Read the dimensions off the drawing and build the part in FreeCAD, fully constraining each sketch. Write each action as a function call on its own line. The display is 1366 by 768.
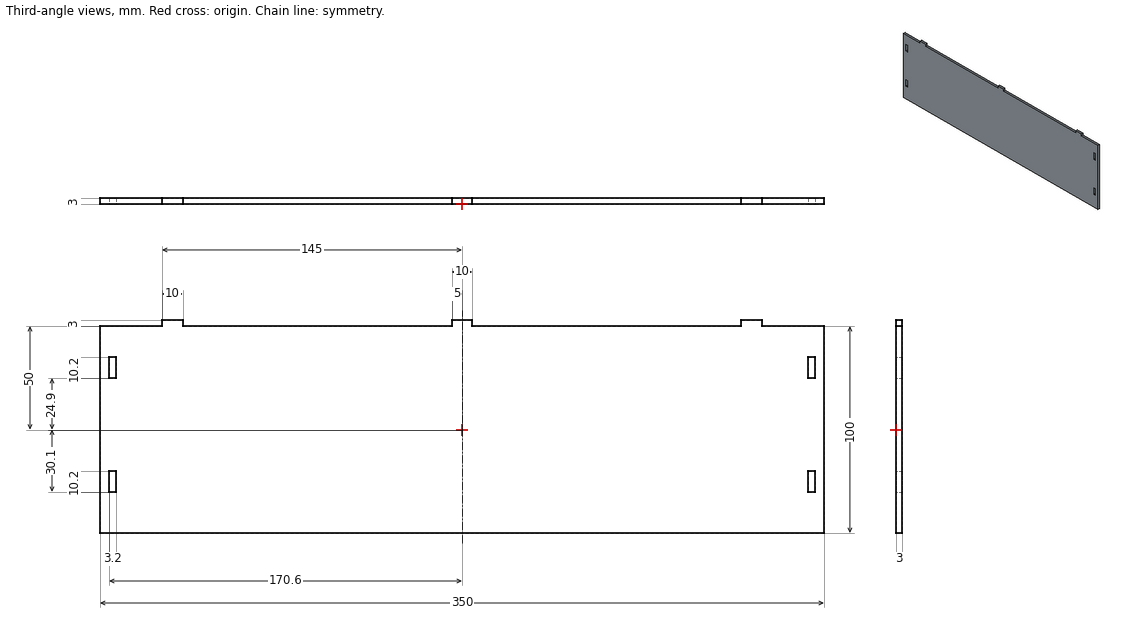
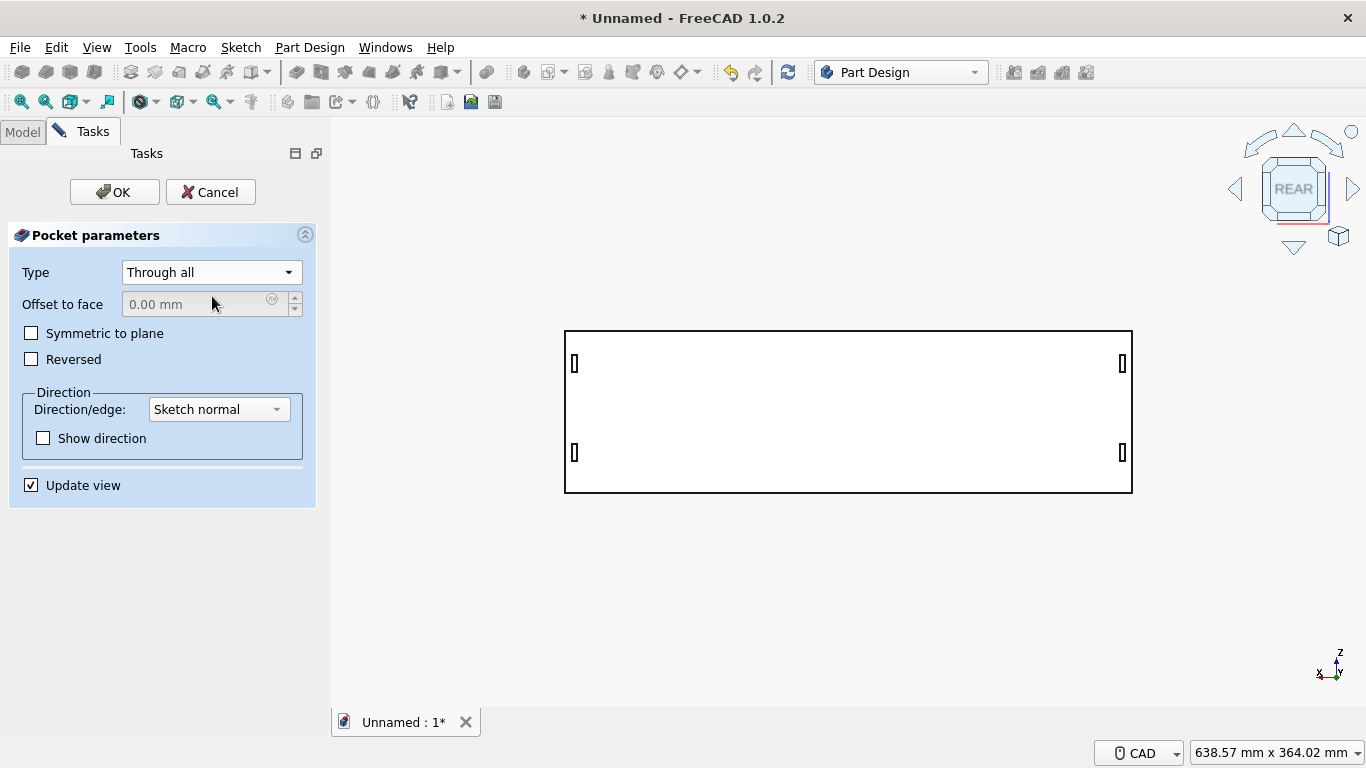
click(115, 192)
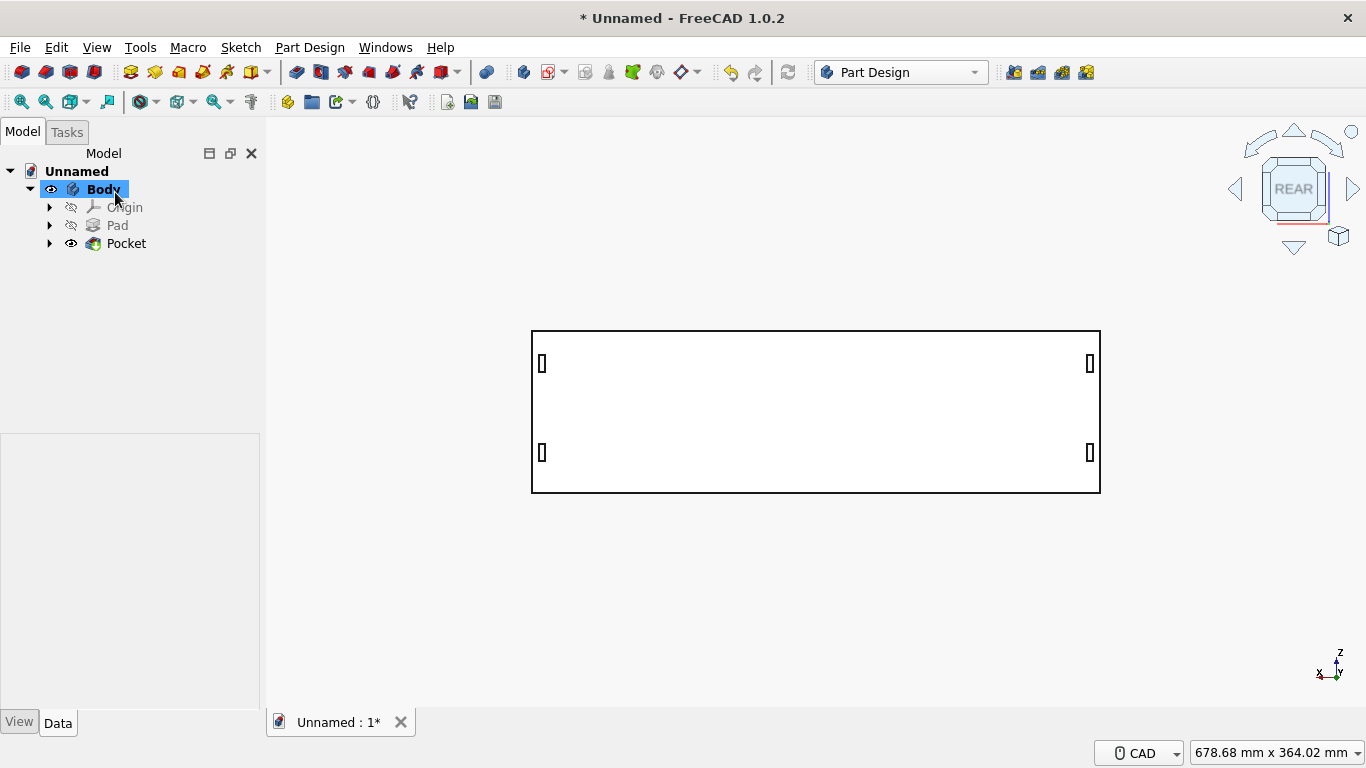
click(654, 411)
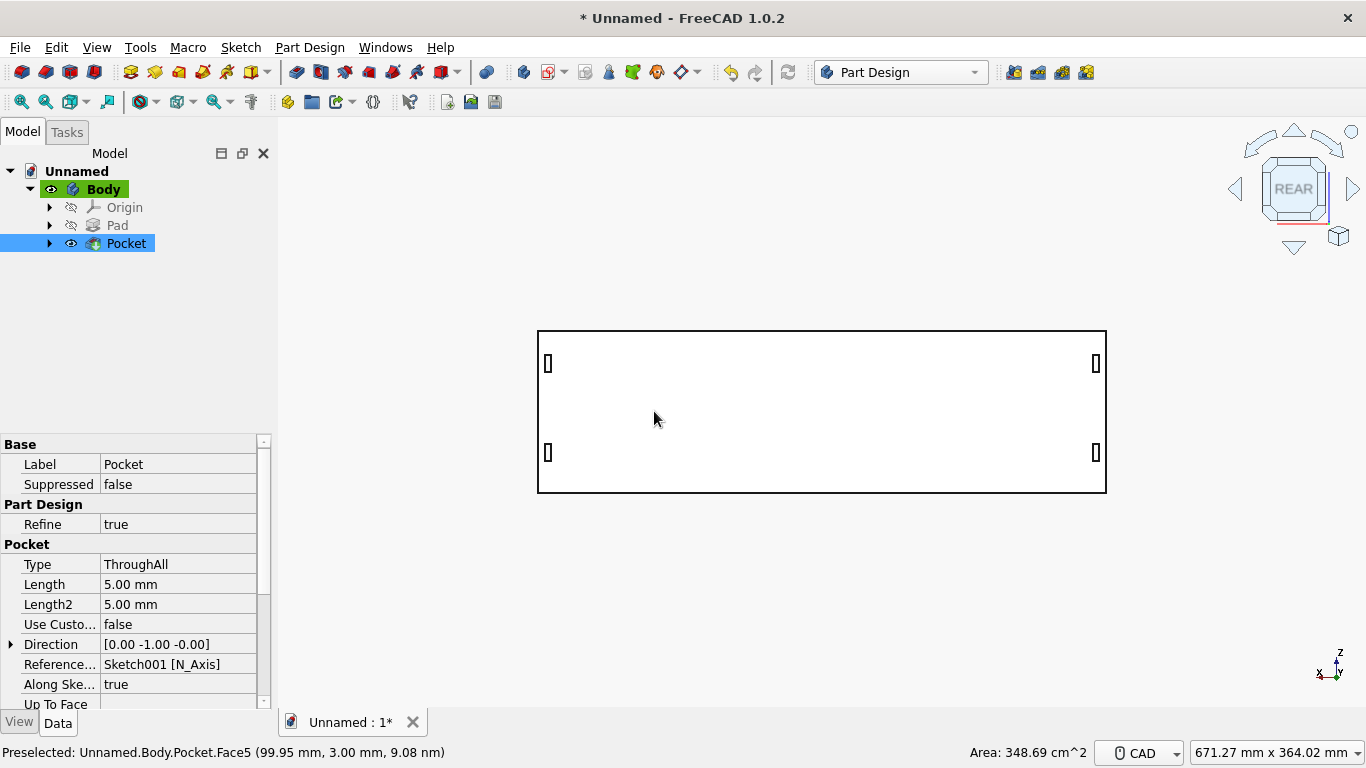
click(548, 72)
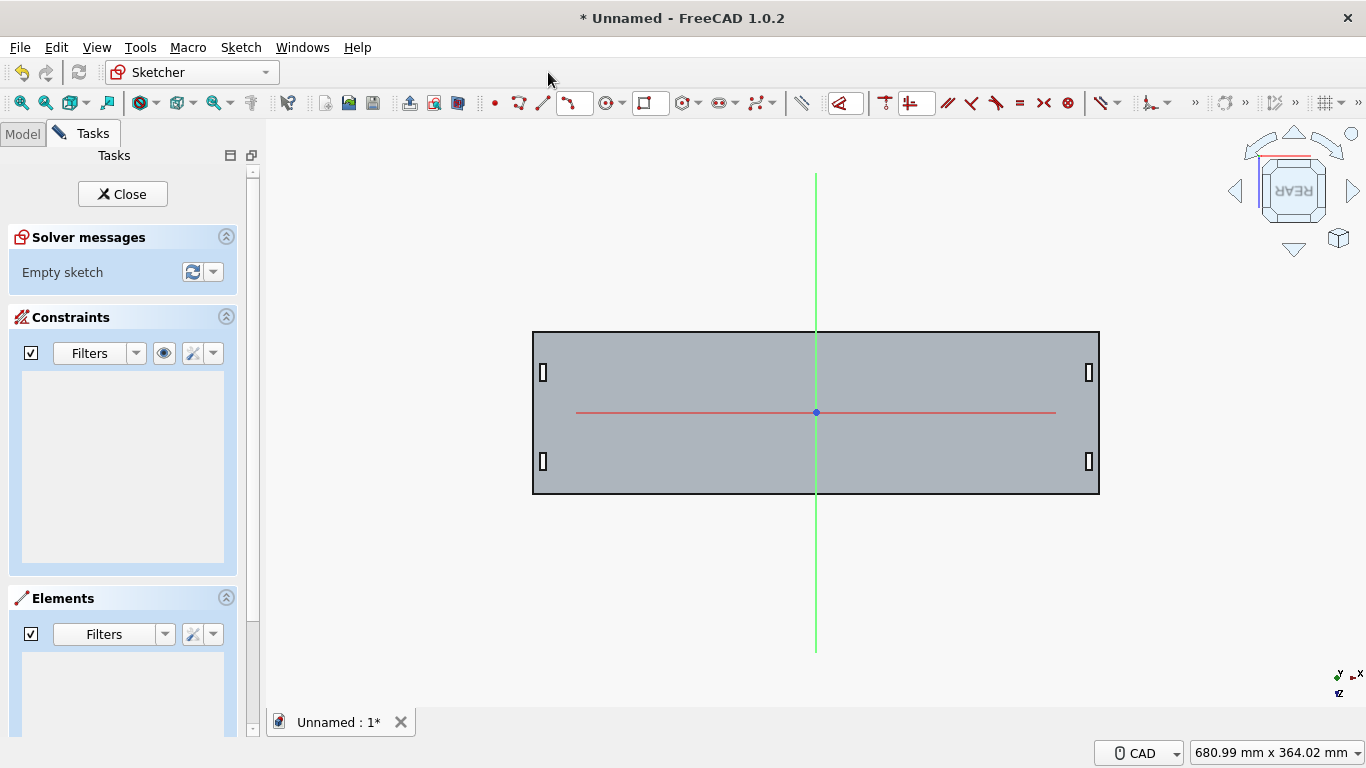
scroll(955, 543, up, 2)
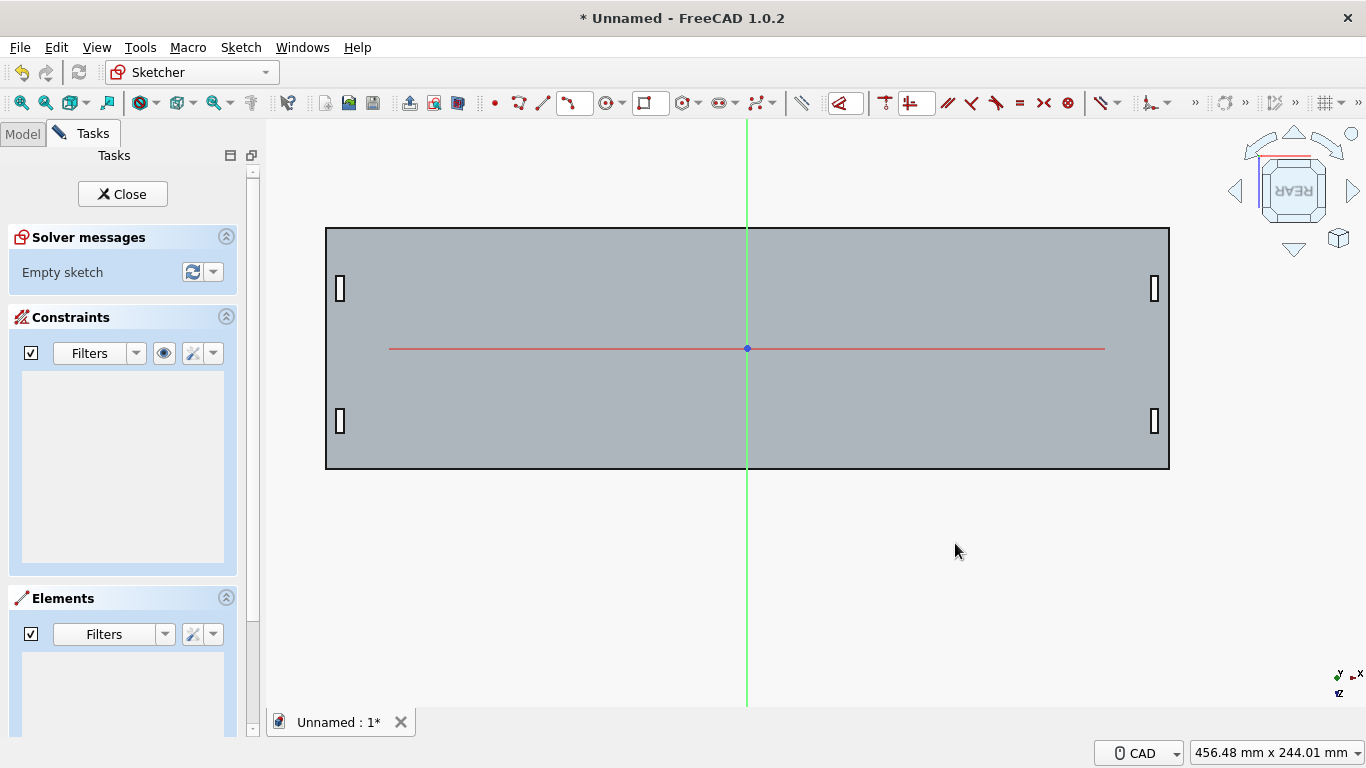
key(g)
key(r)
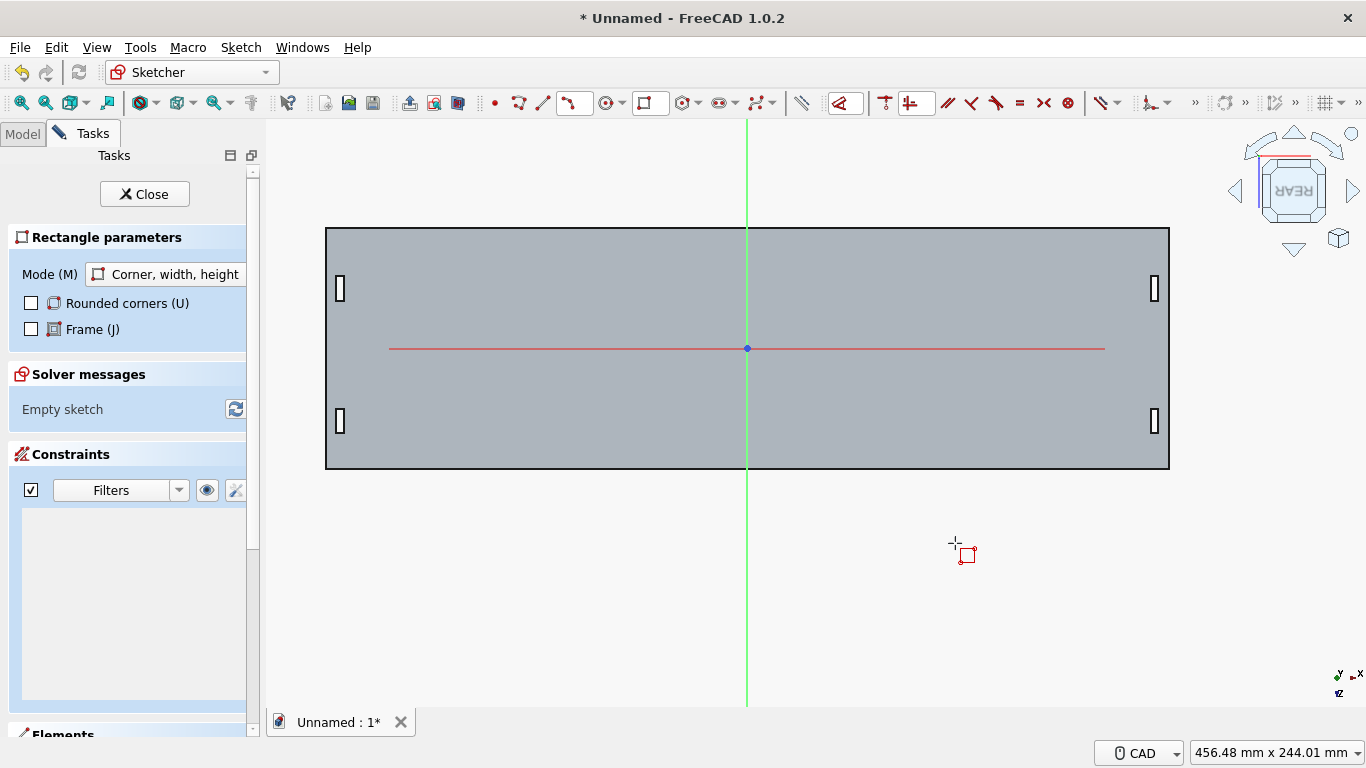
scroll(398, 469, up, 4)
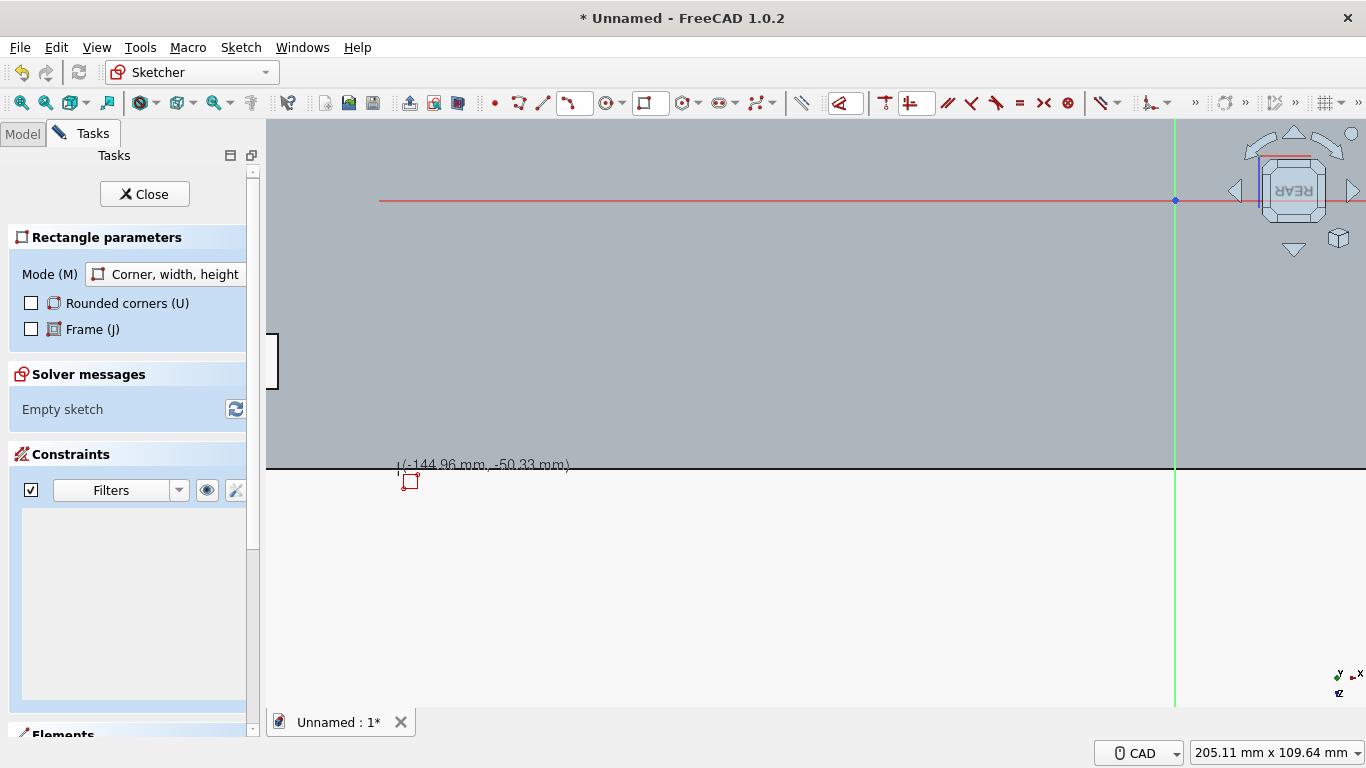
click(398, 469)
click(451, 485)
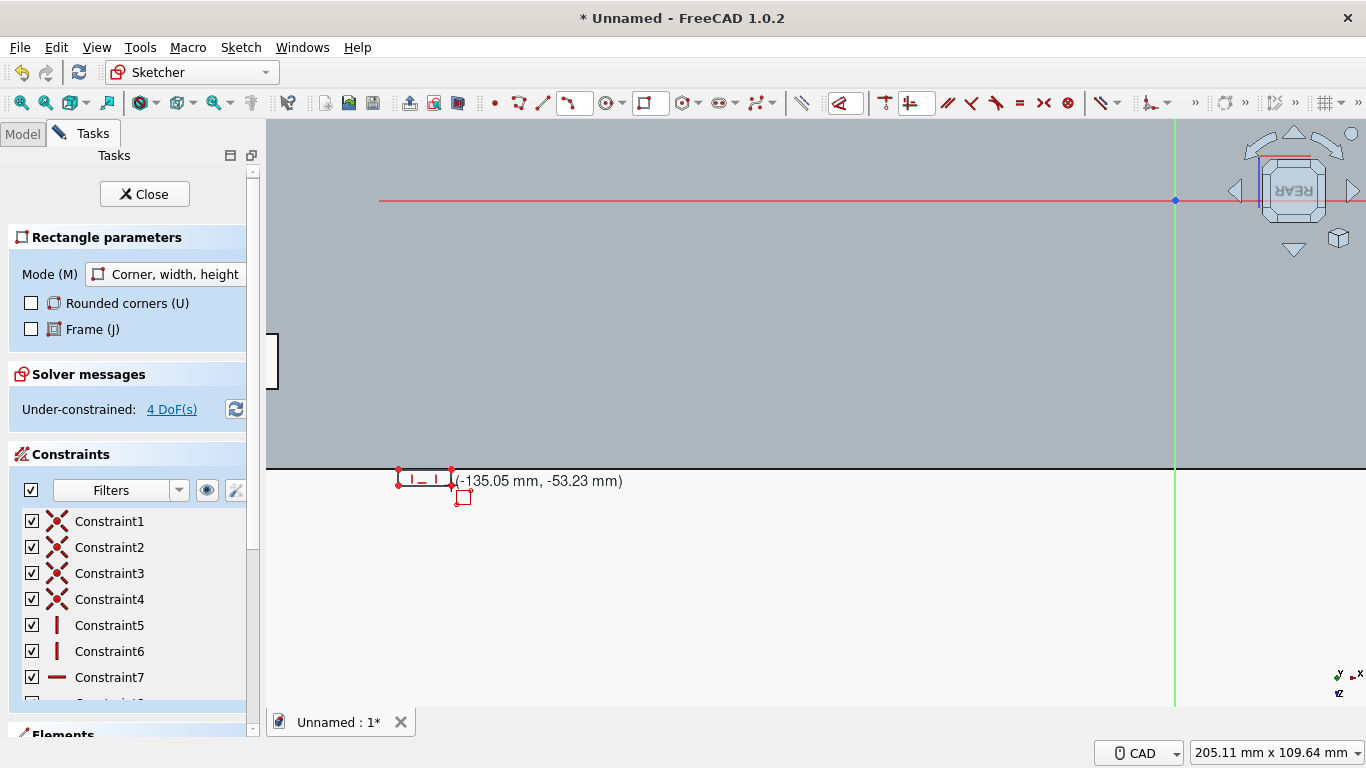
click(1148, 469)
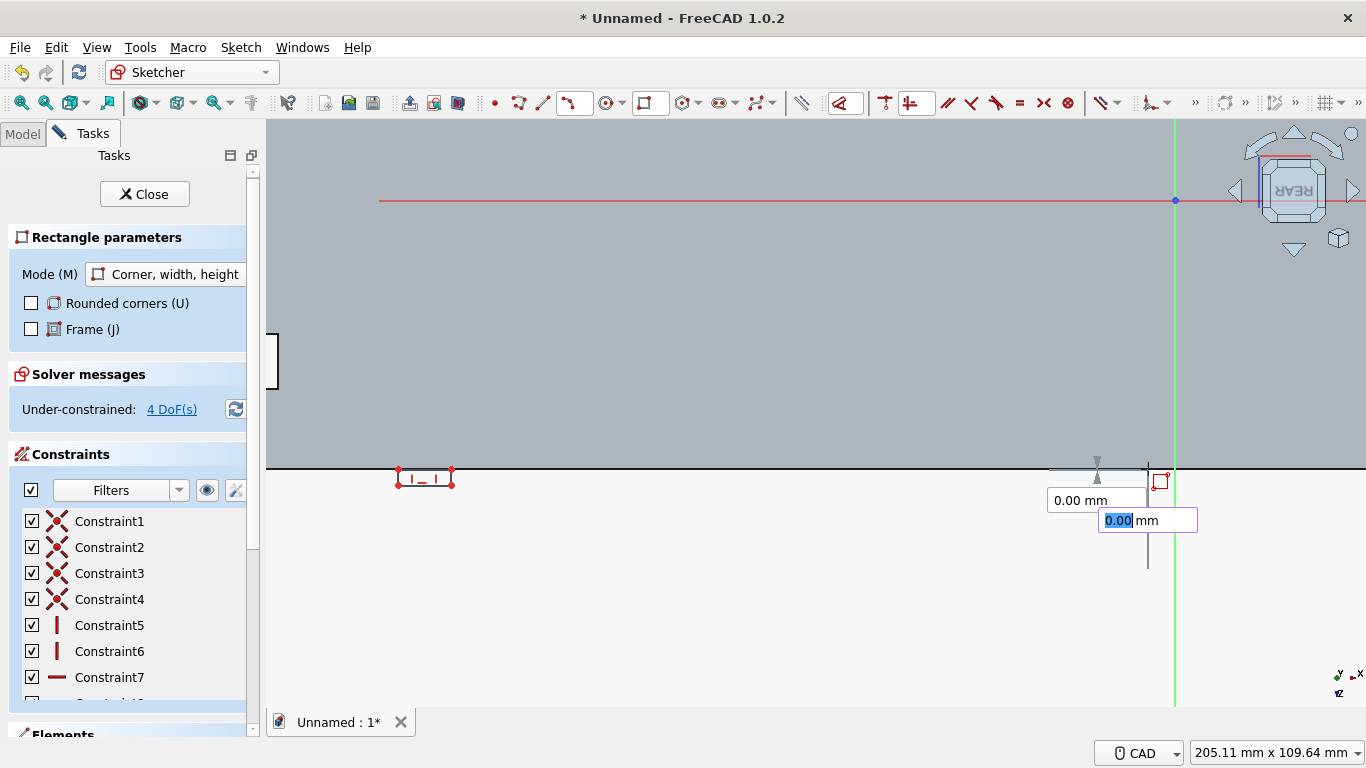
scroll(398, 470, down, 4)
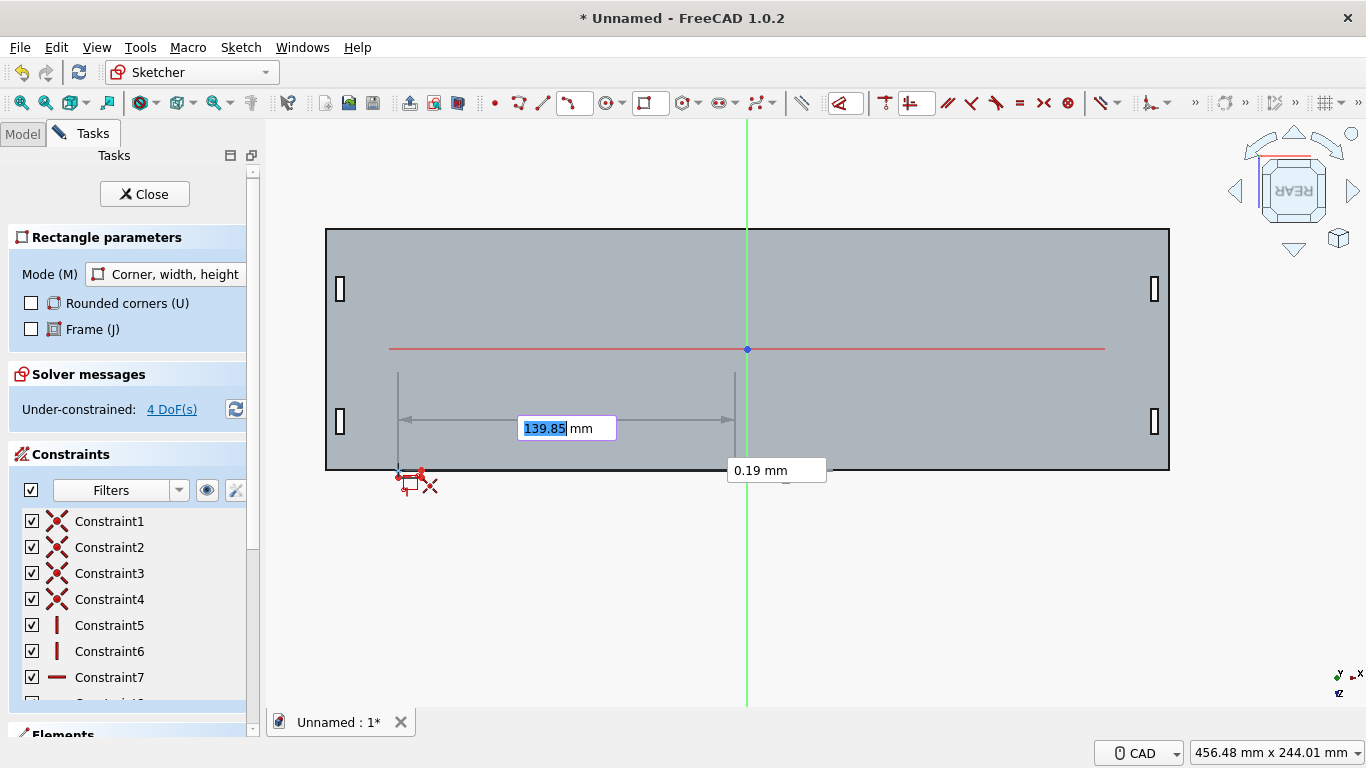
scroll(759, 477, up, 2)